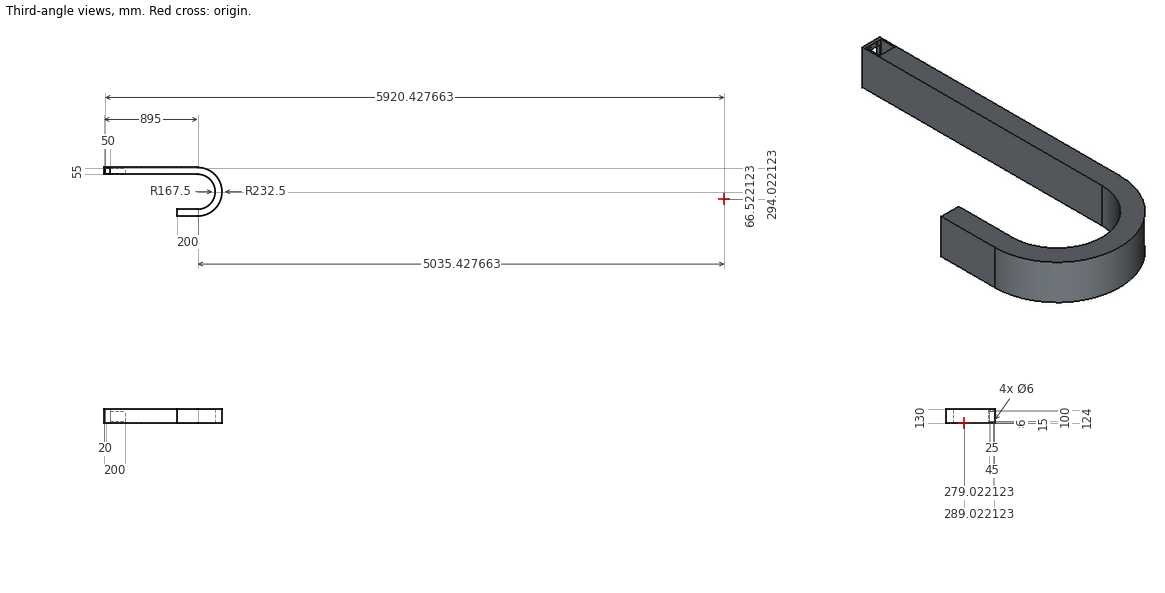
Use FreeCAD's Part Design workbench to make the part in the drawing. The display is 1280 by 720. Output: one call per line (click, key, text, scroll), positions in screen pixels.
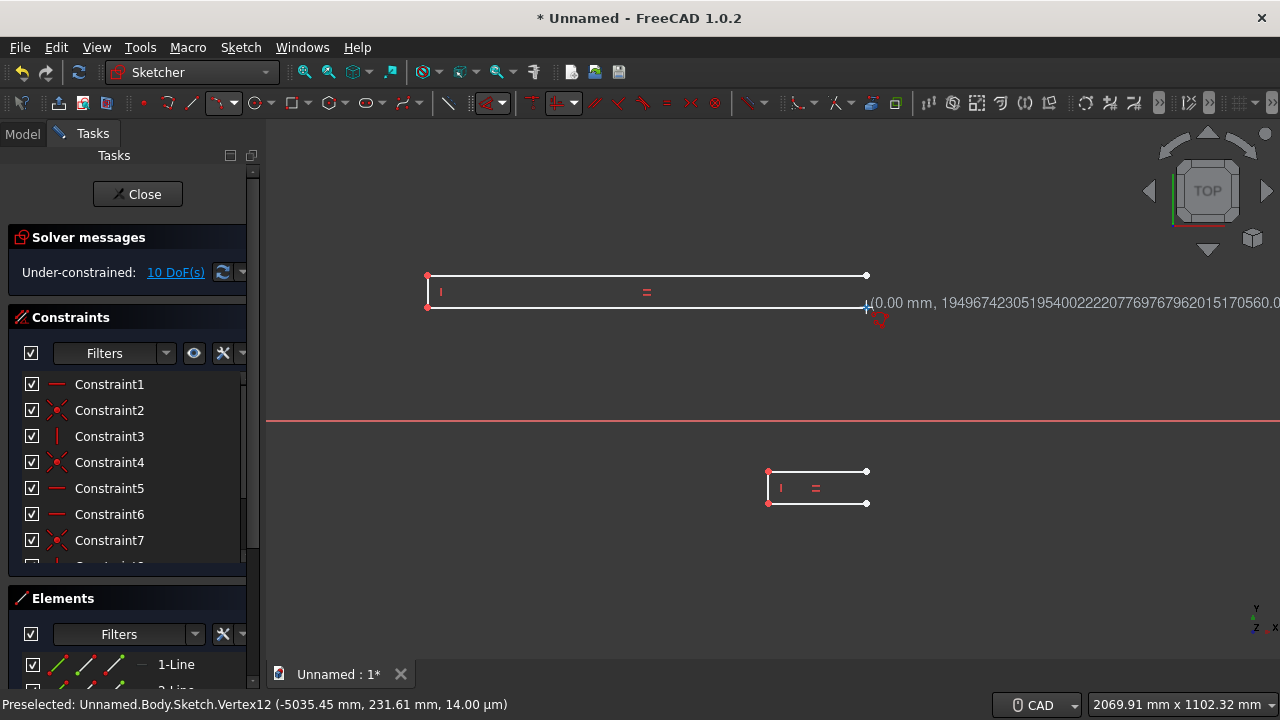
click(218, 104)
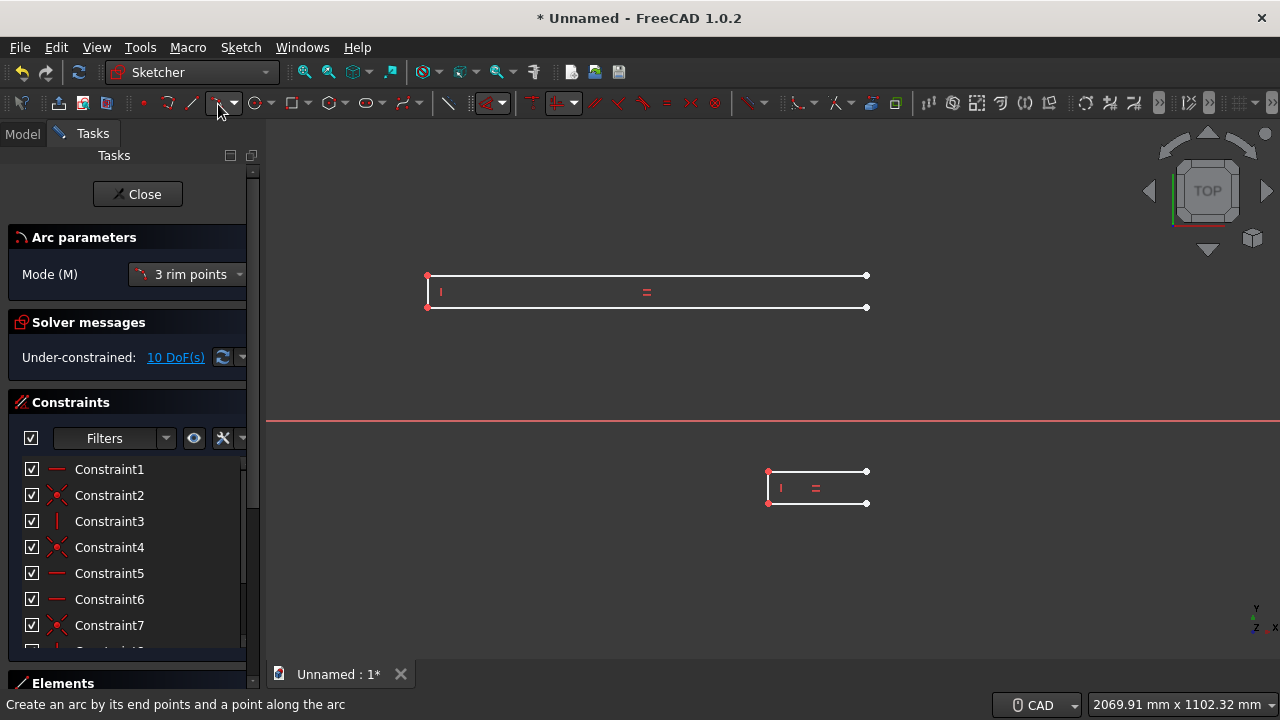
click(866, 504)
click(866, 276)
click(980, 389)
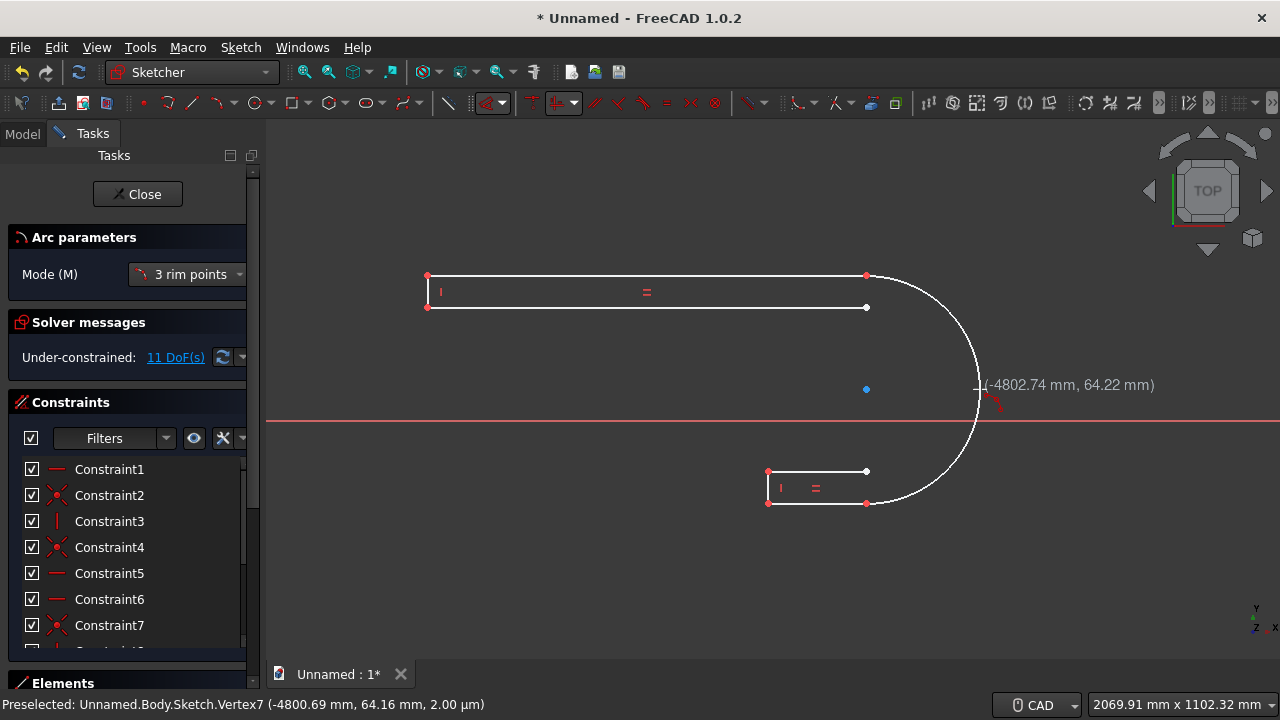
click(866, 308)
click(866, 472)
click(948, 389)
key(Escape)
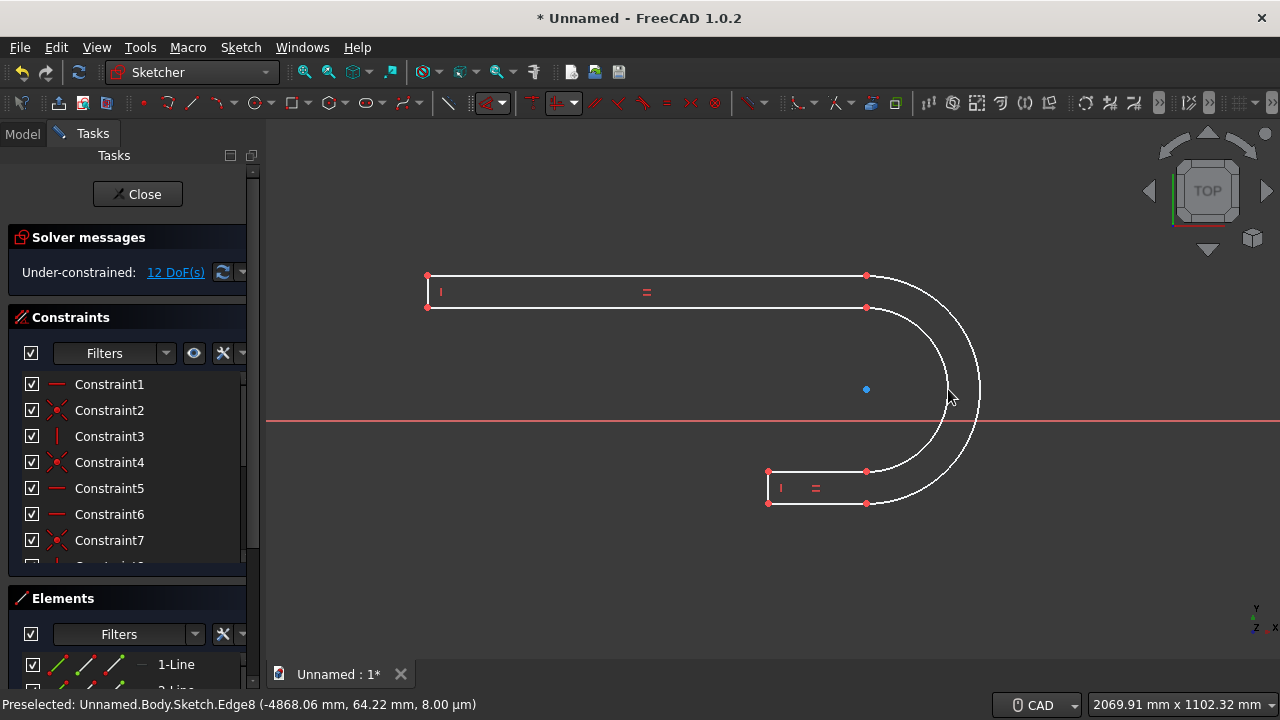
click(958, 457)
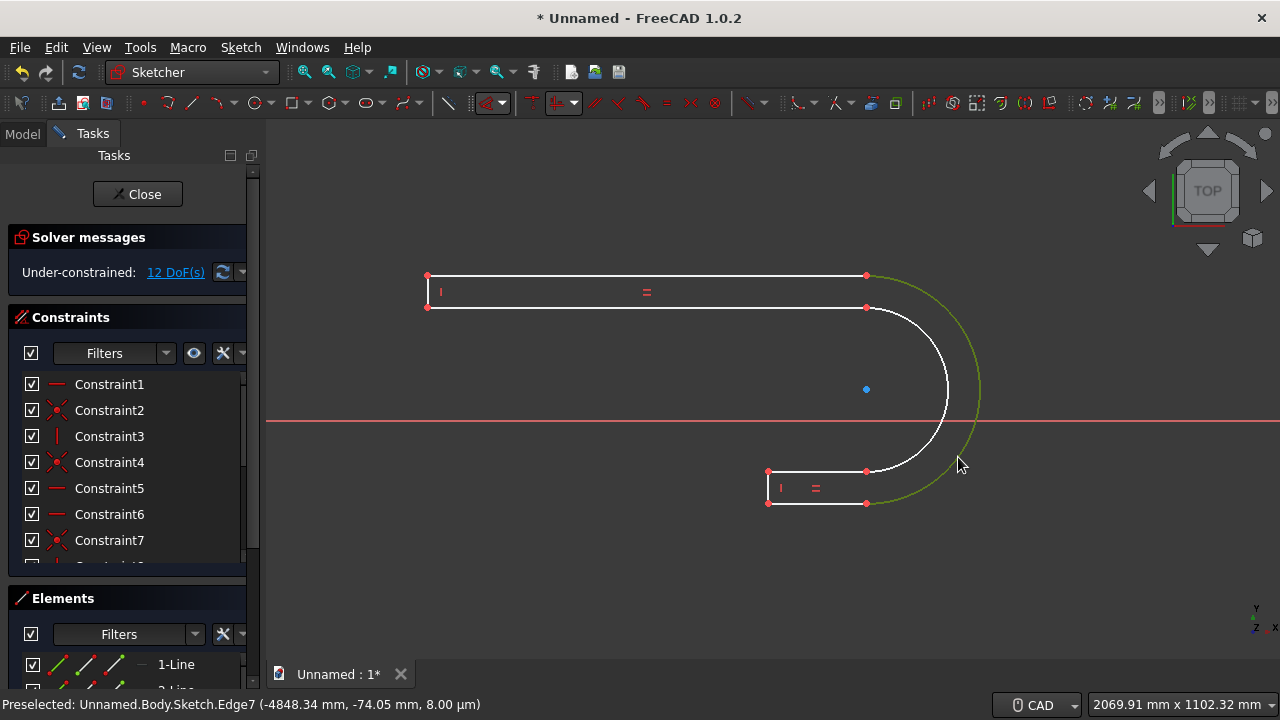
click(932, 438)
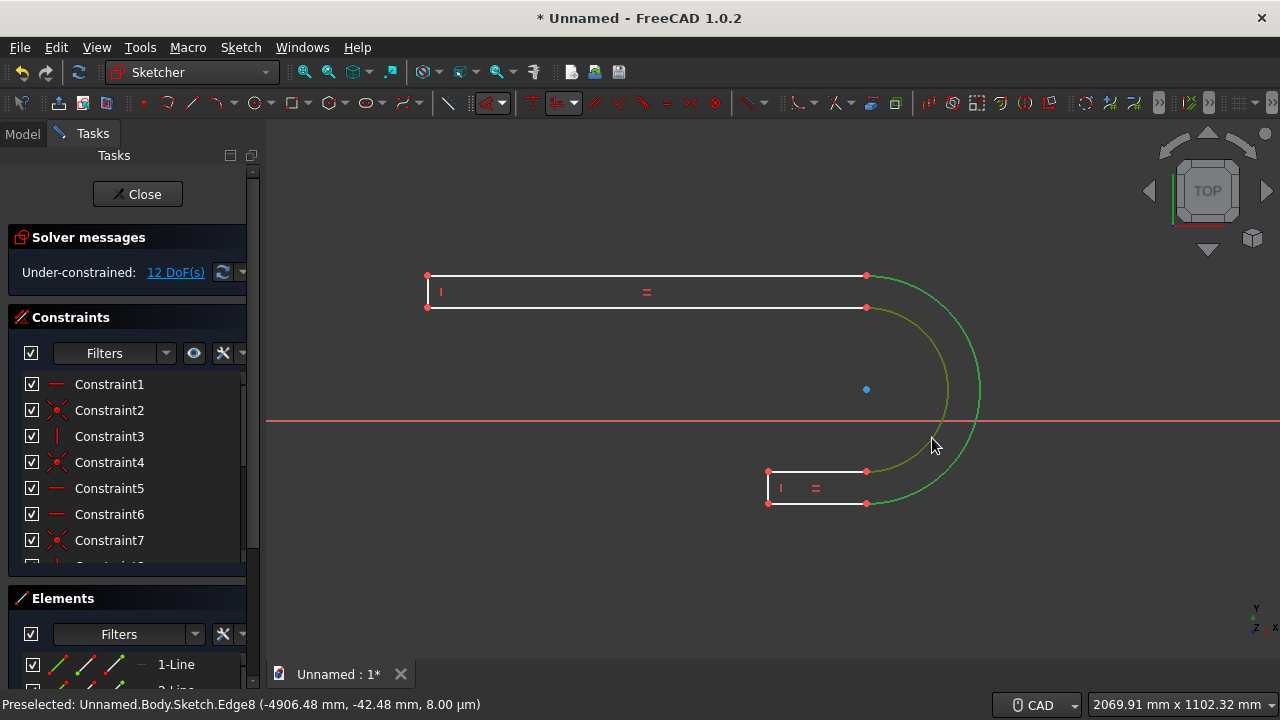
key(c)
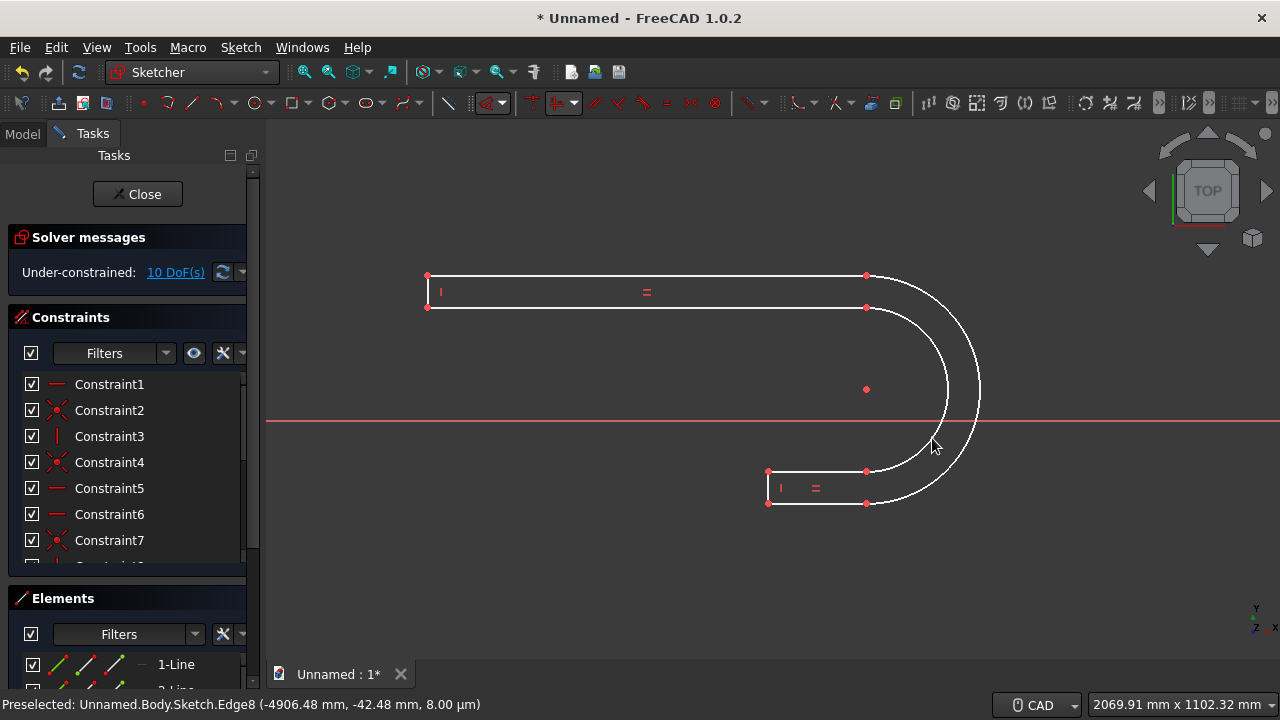
click(958, 457)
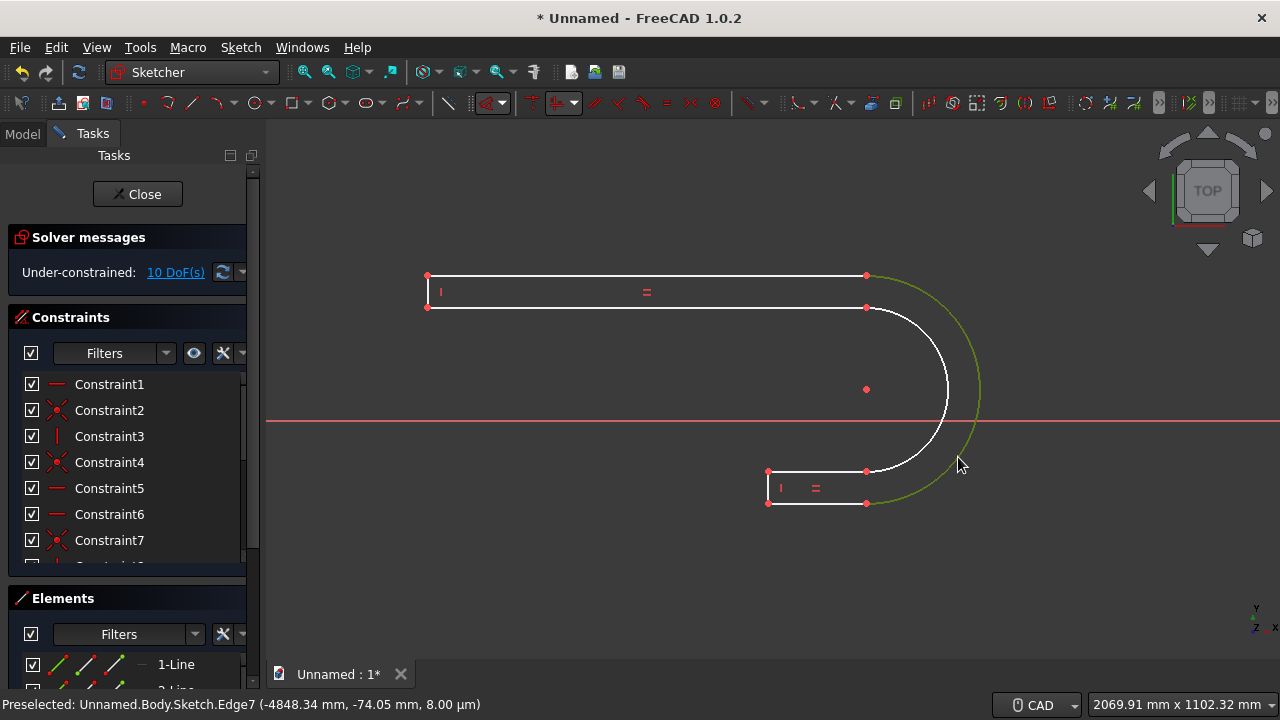
key(k)
key(r)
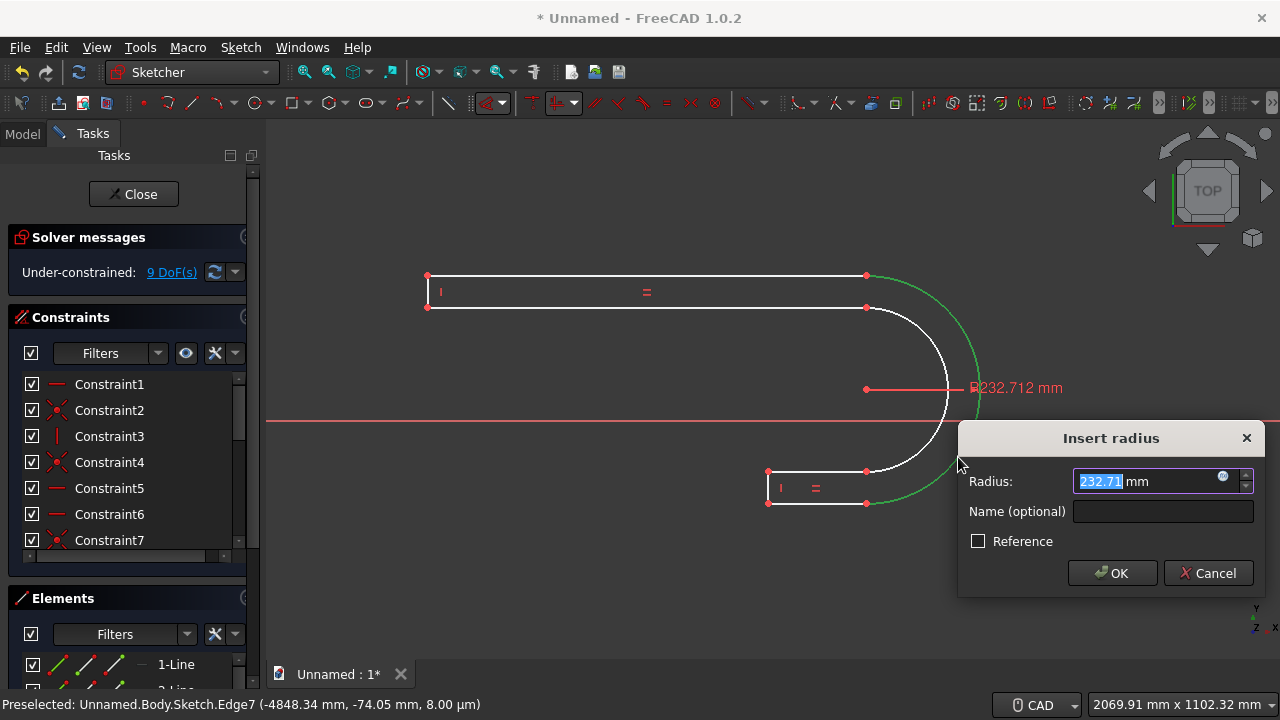
text(232.5)
key(Return)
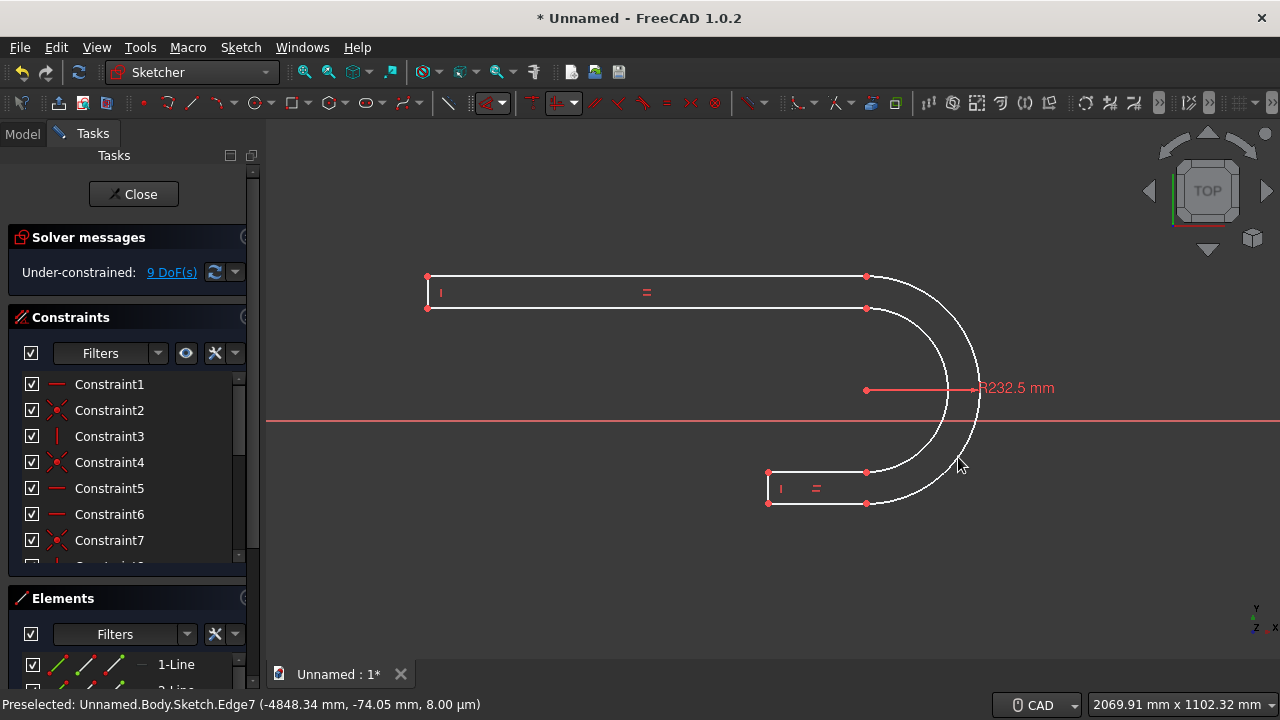
click(932, 438)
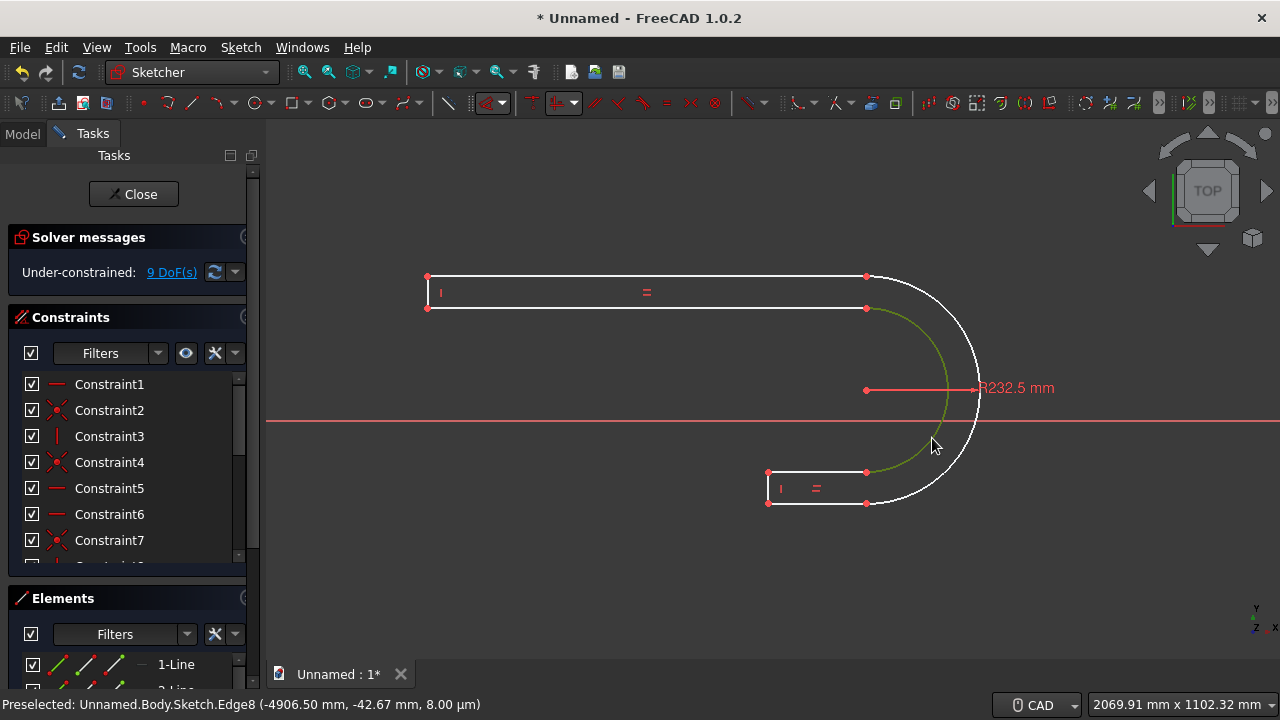
key(k)
key(r)